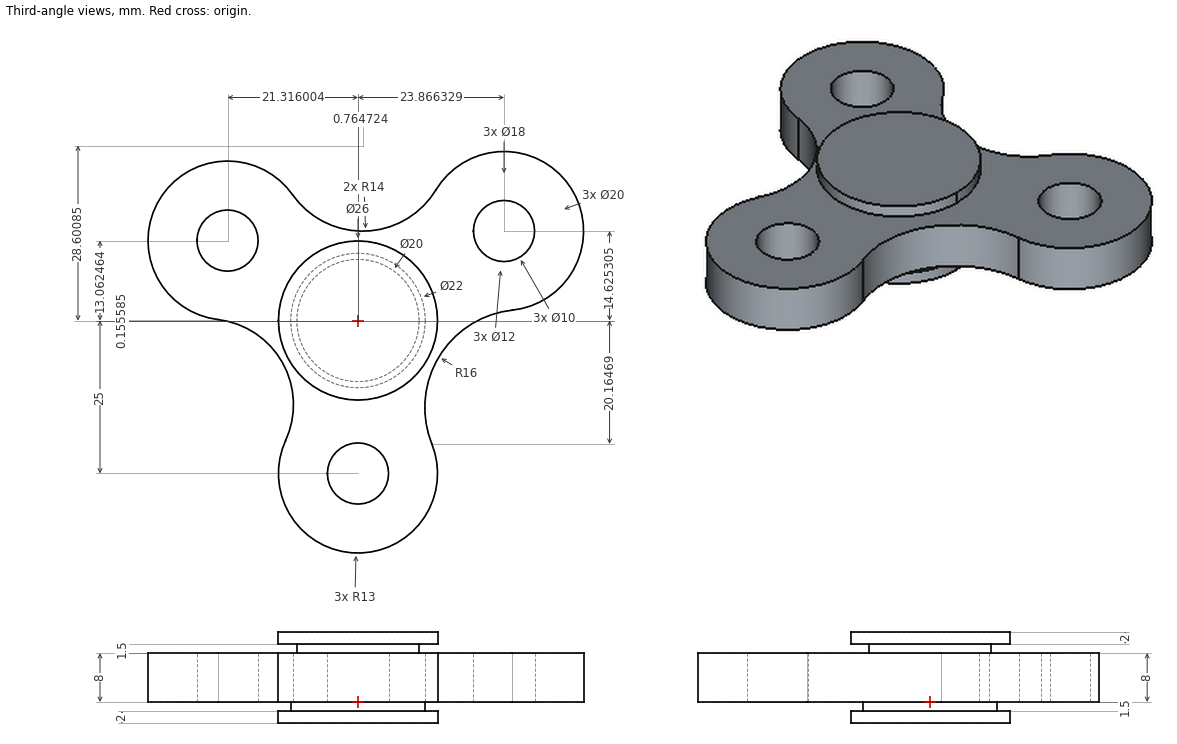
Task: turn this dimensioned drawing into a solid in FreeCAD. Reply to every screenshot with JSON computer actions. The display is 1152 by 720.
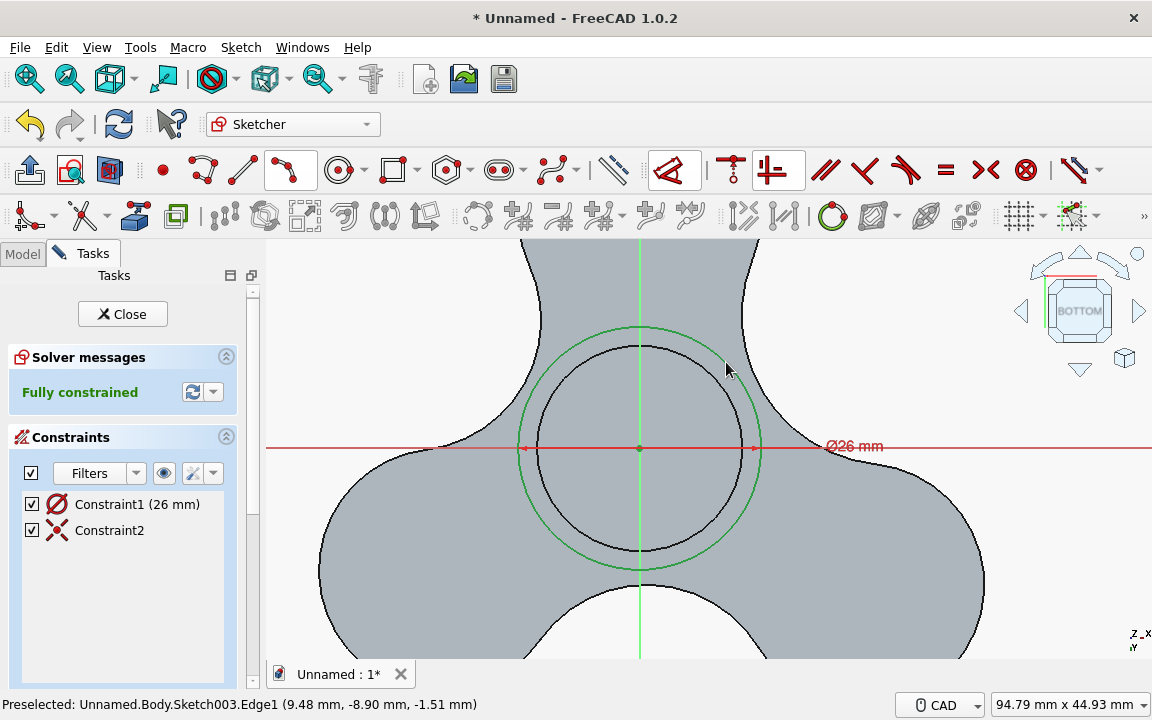
{"action": "left_click", "coordinate": [123, 314]}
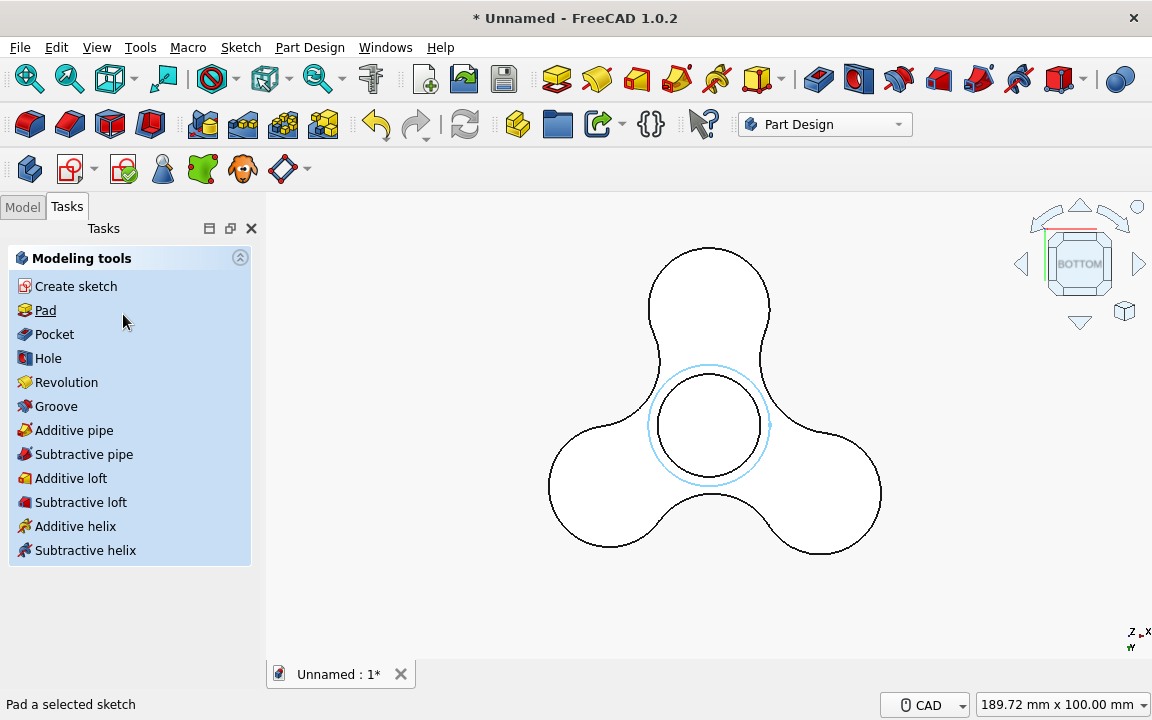
{"action": "left_click", "coordinate": [558, 80]}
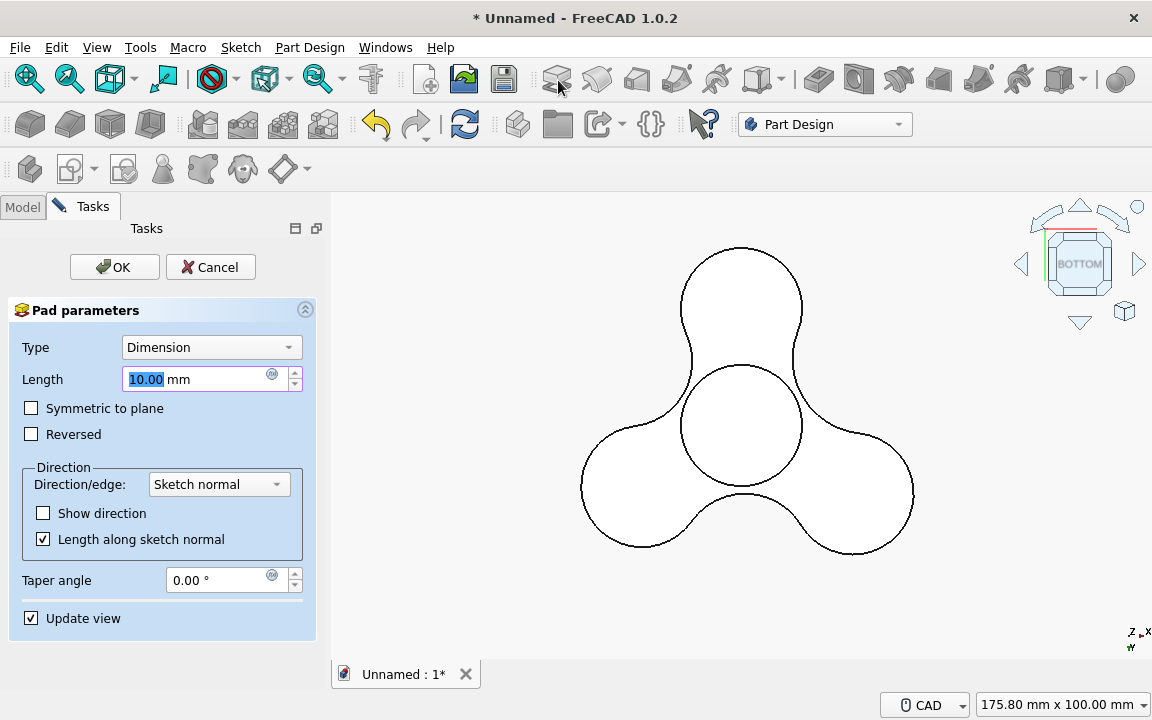
{"action": "type", "text": "2"}
{"action": "key", "text": "Tab"}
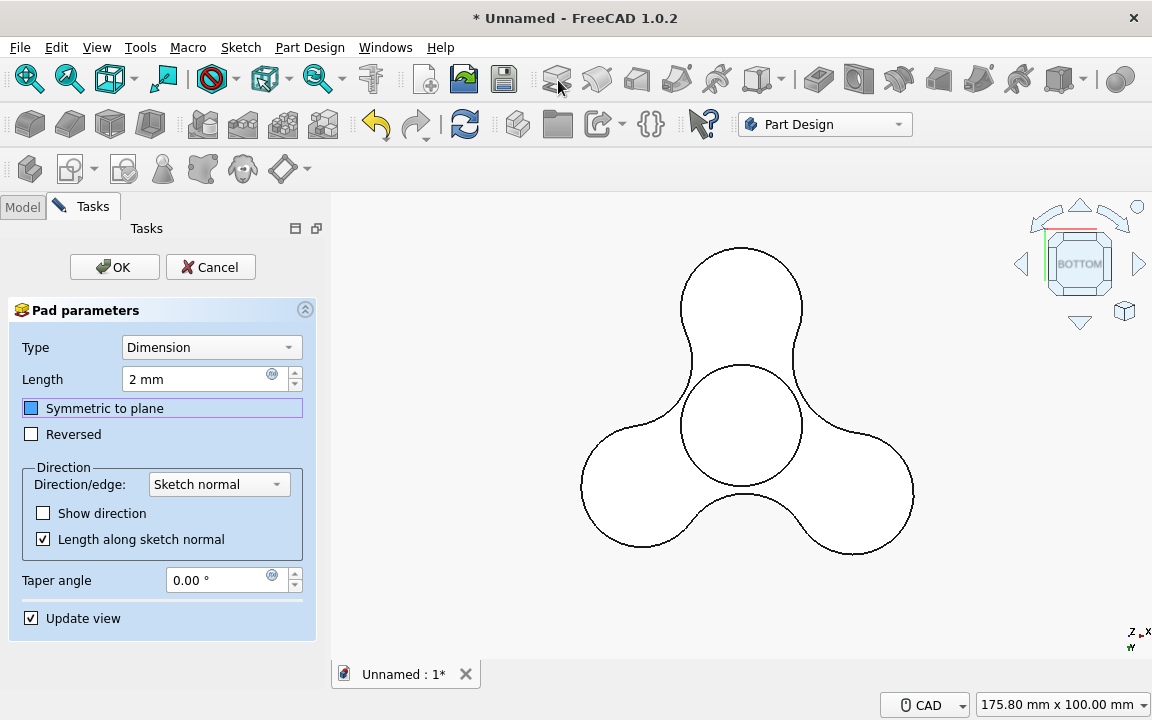
{"action": "left_click", "coordinate": [115, 267]}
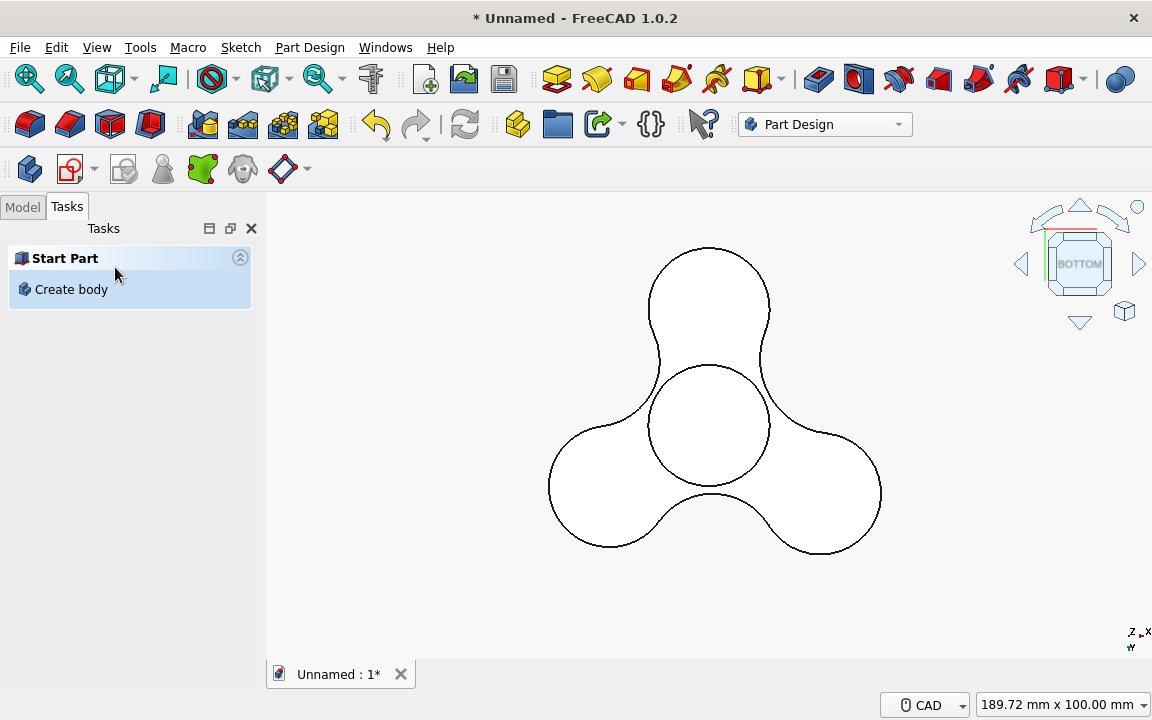
{"action": "left_click", "coordinate": [23, 206]}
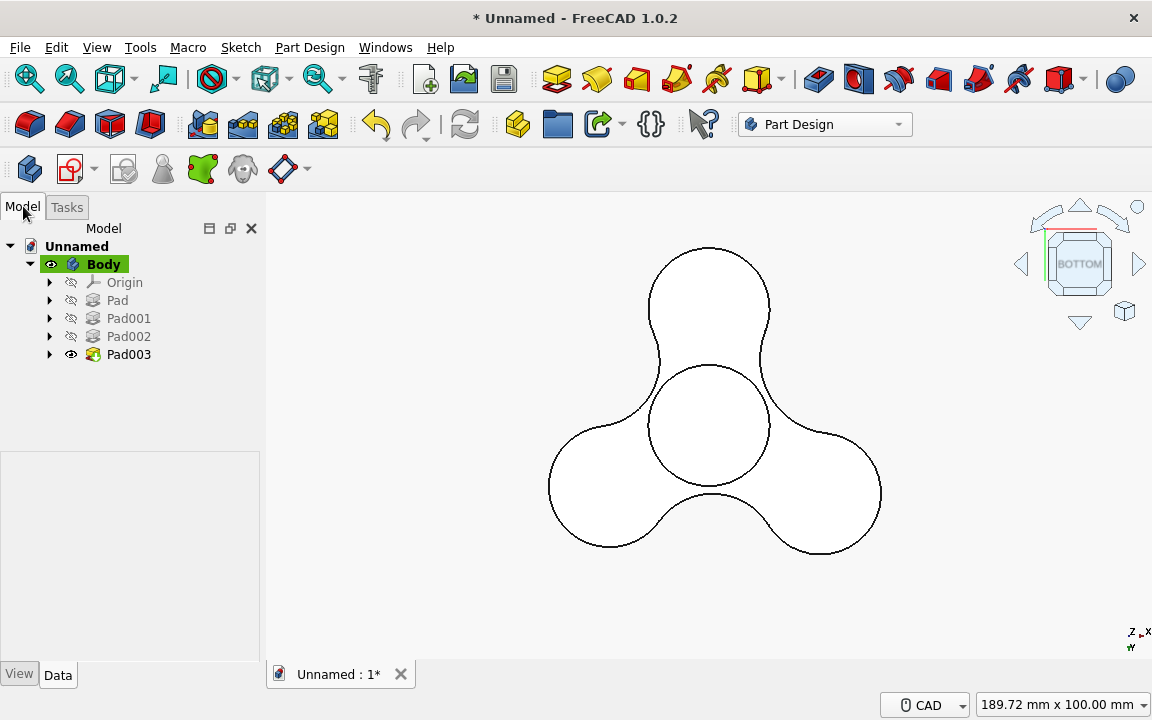
{"action": "left_click", "coordinate": [50, 282]}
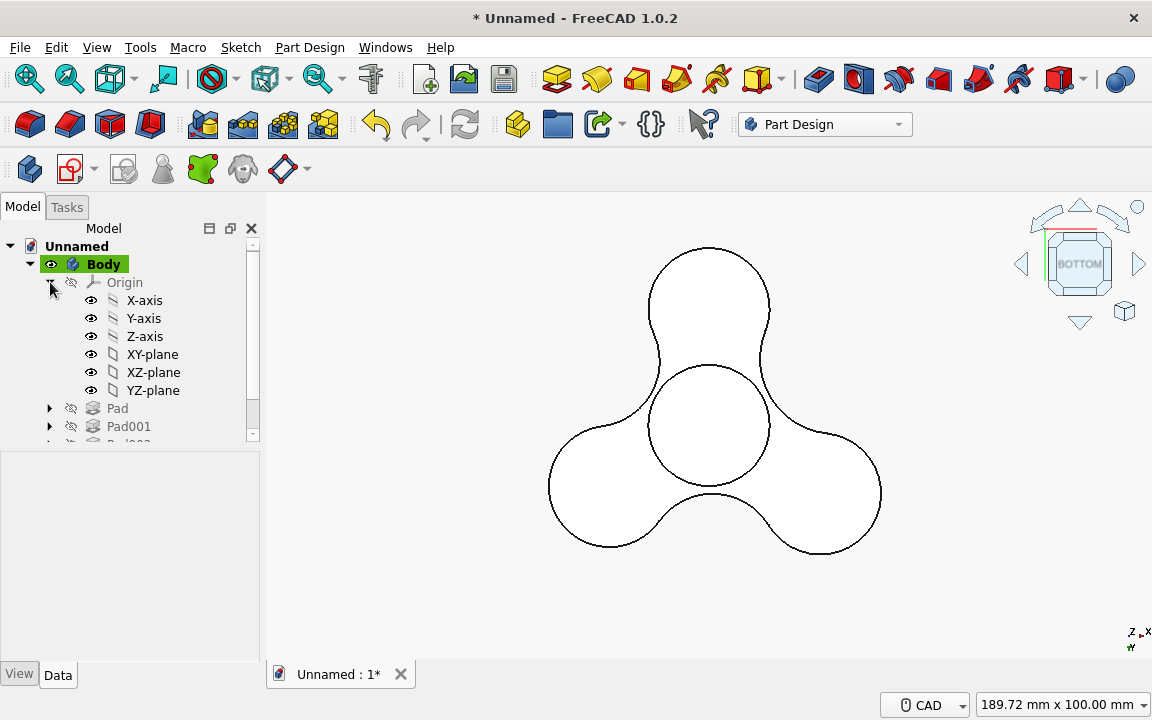
{"action": "left_click", "coordinate": [136, 354]}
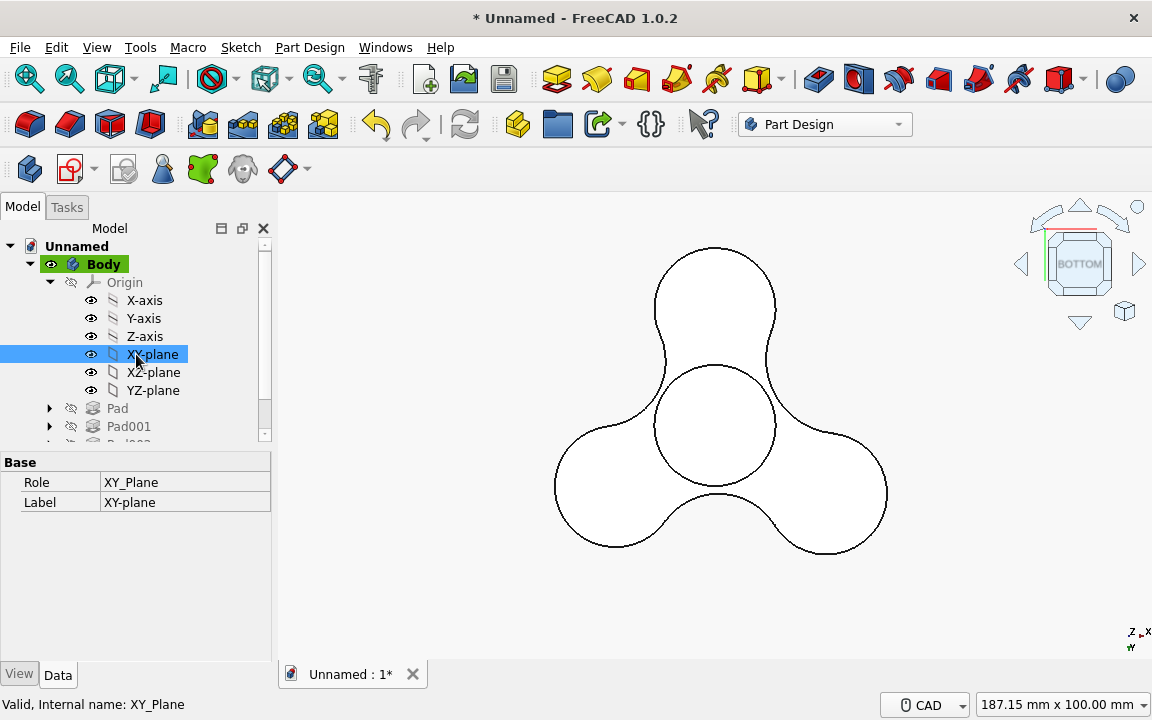
{"action": "left_click", "coordinate": [284, 170]}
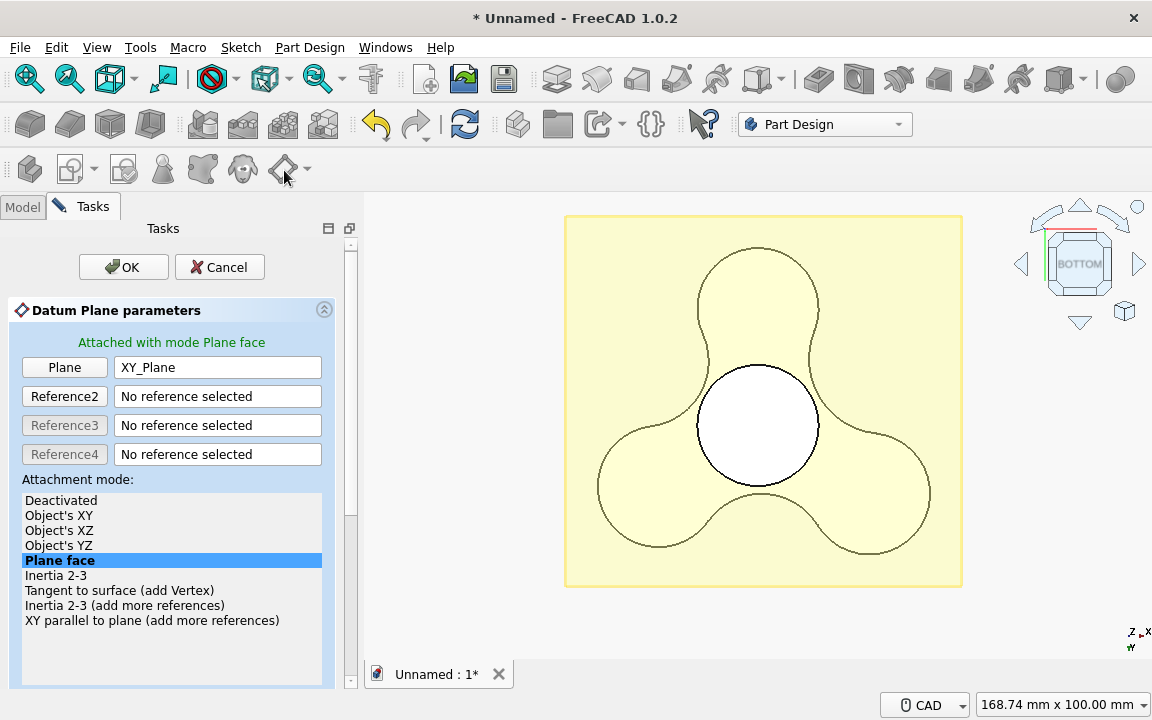
{"action": "scroll", "coordinate": [351, 463], "scroll_direction": "down", "scroll_amount": 3}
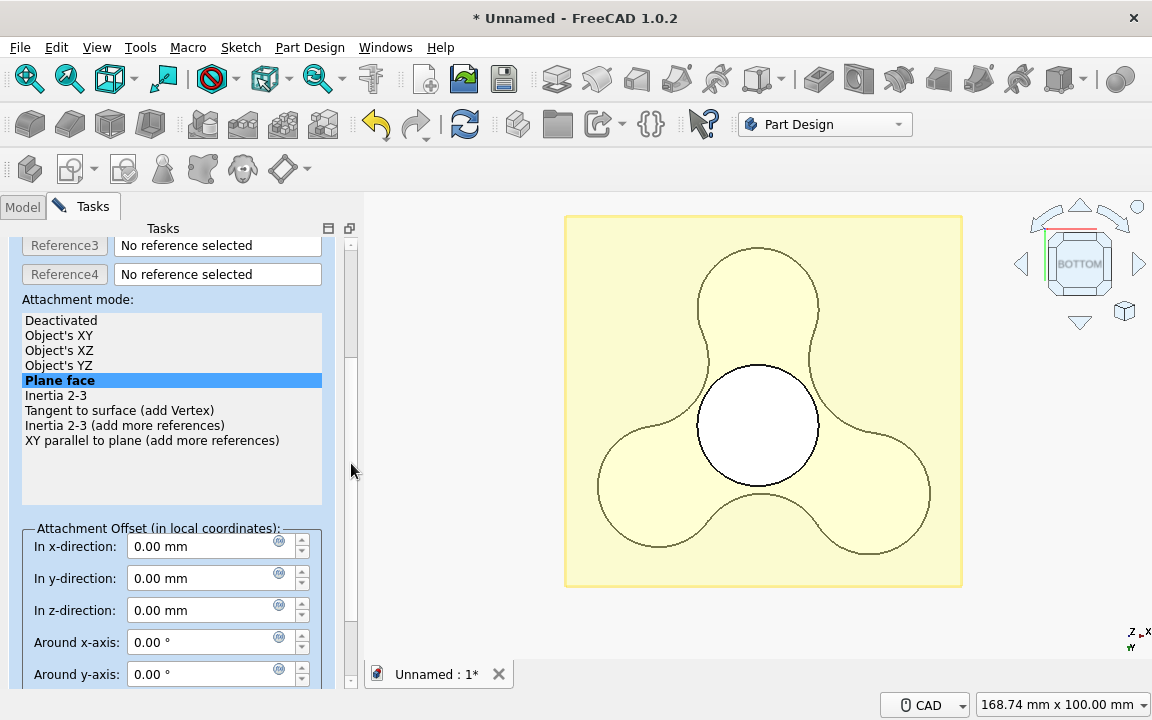
{"action": "triple_click", "coordinate": [210, 610]}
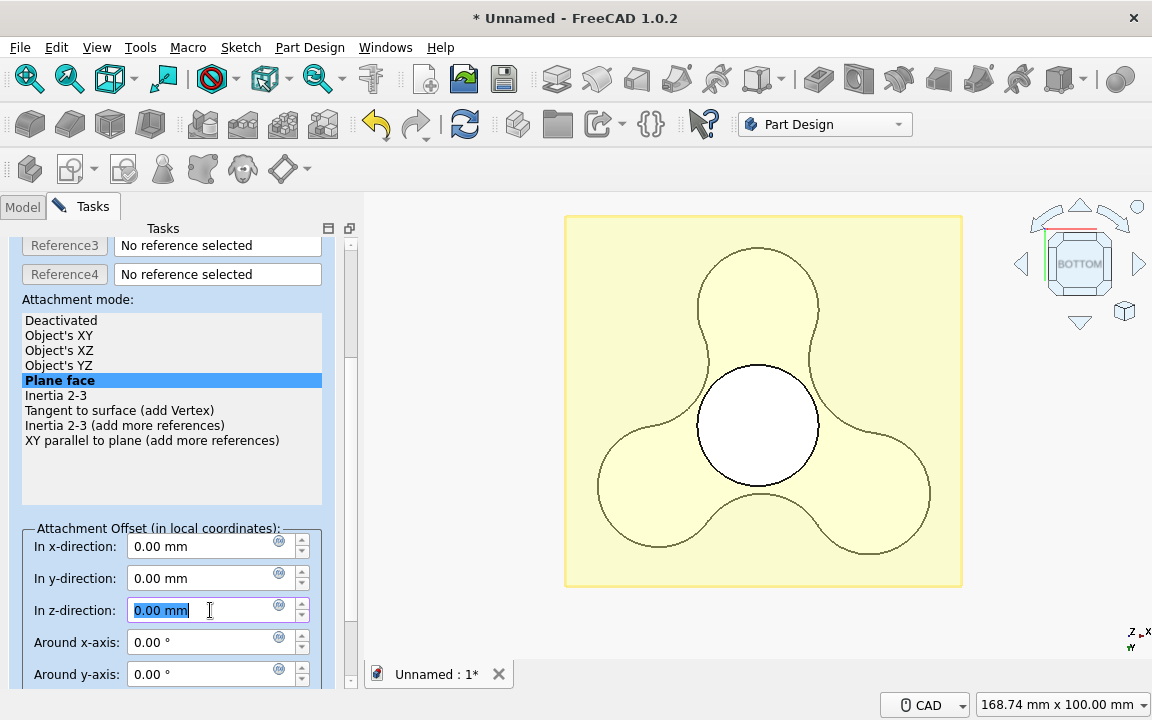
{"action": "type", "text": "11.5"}
{"action": "key", "text": "Tab"}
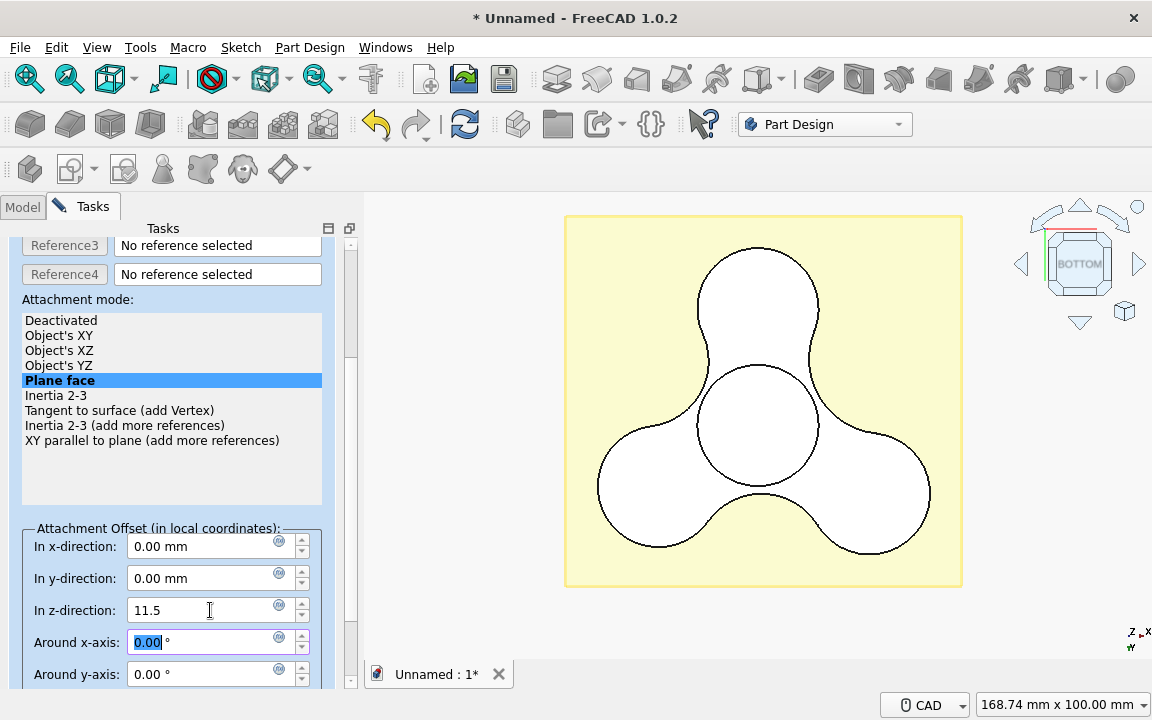
{"action": "scroll", "coordinate": [351, 463], "scroll_direction": "up", "scroll_amount": 4}